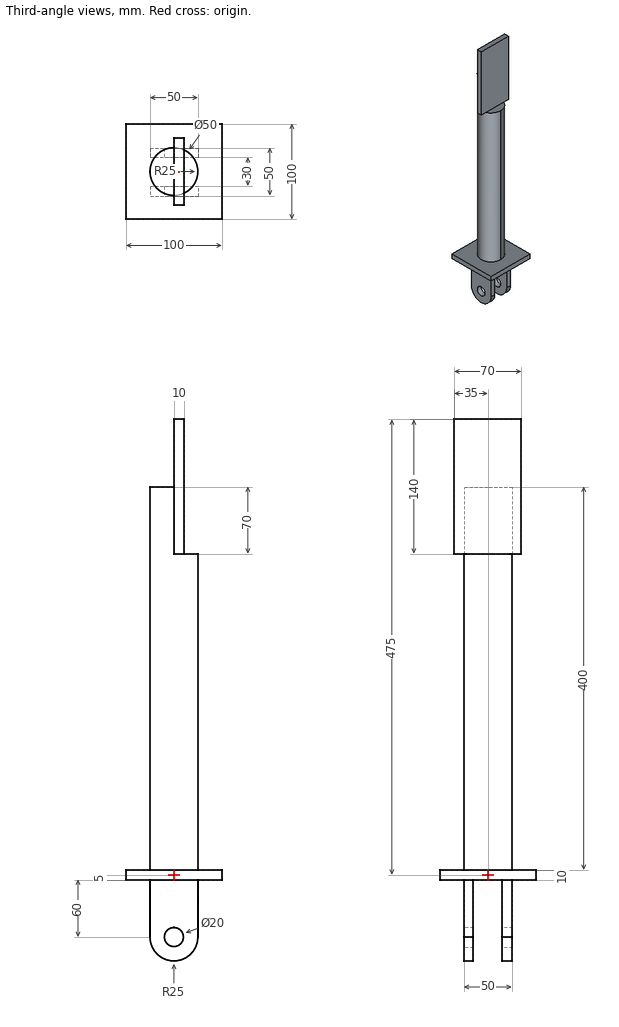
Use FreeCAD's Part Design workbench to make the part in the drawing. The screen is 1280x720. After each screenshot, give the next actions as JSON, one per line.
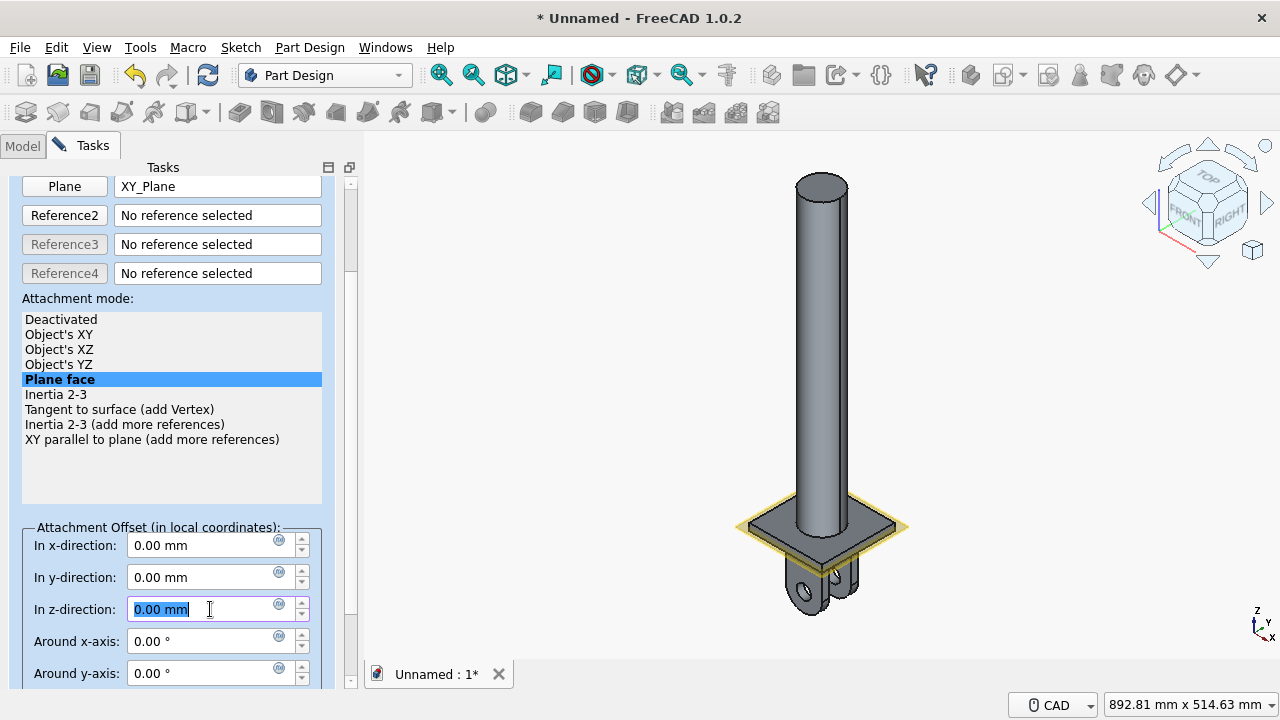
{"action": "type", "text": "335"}
{"action": "key", "text": "Tab"}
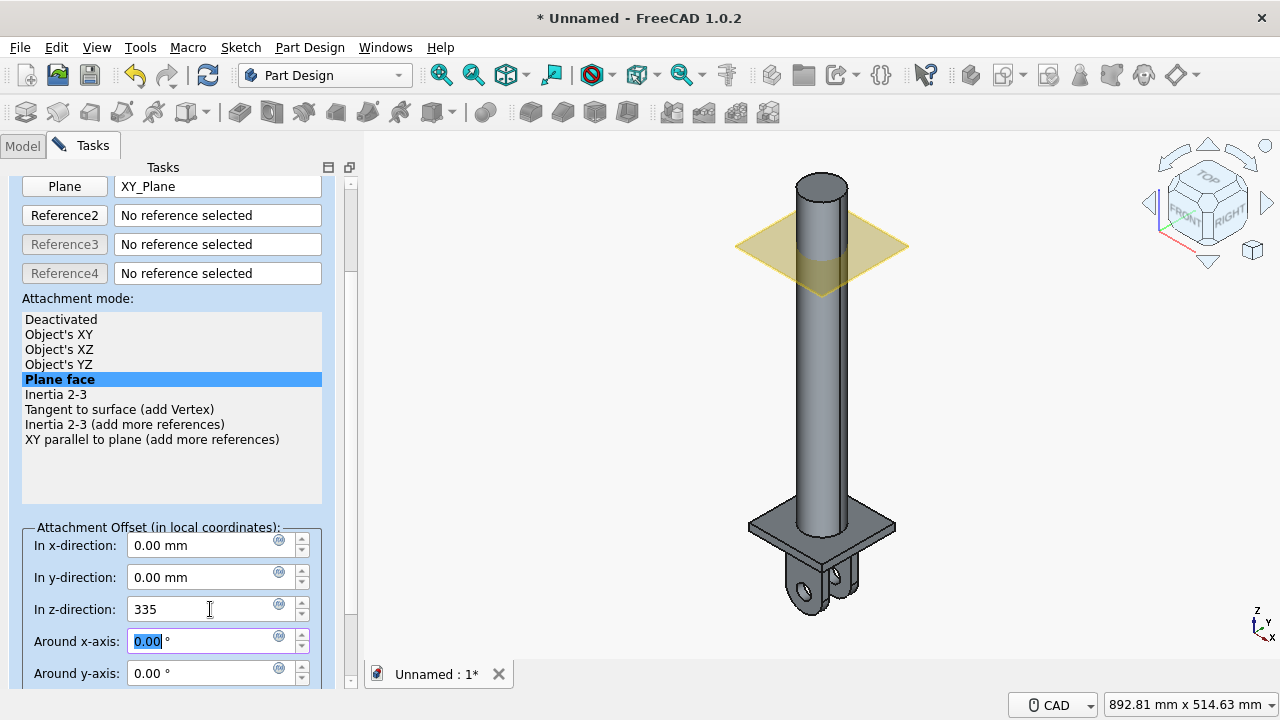
{"action": "scroll", "coordinate": [351, 432], "scroll_direction": "up", "scroll_amount": 3}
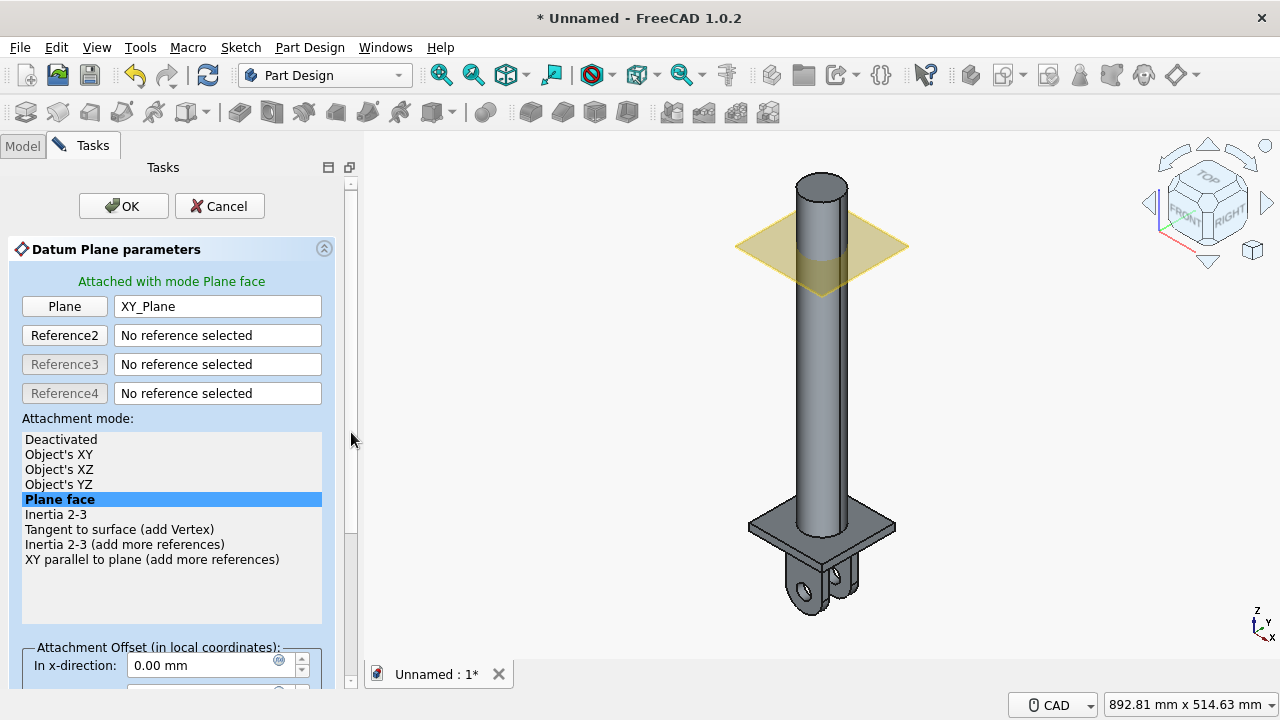
{"action": "left_click", "coordinate": [124, 206]}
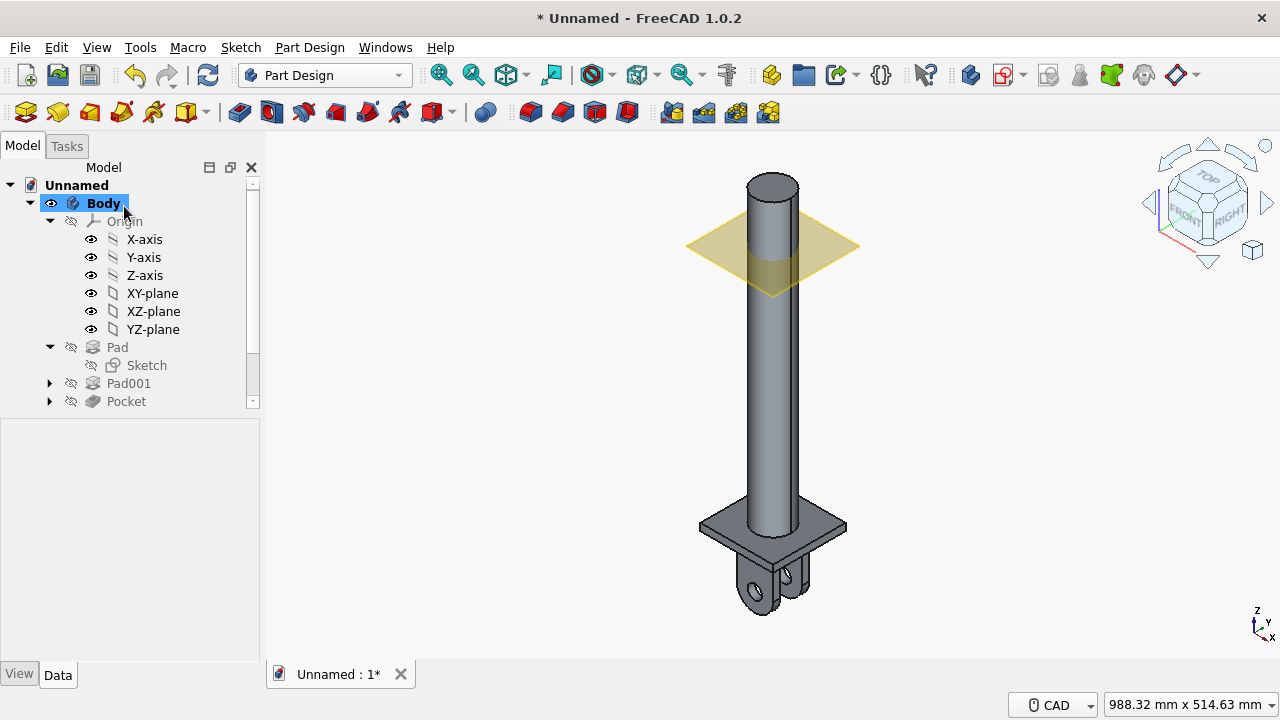
{"action": "scroll", "coordinate": [100, 289], "scroll_direction": "down", "scroll_amount": 3}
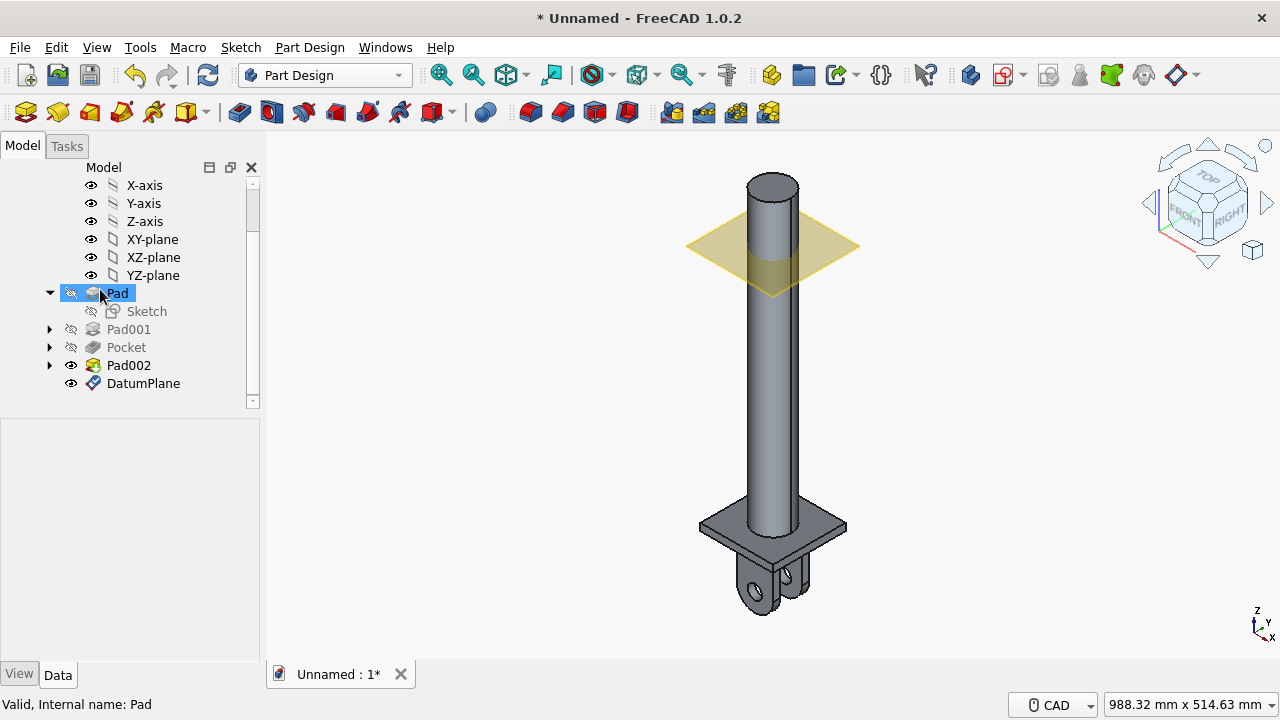
{"action": "left_click", "coordinate": [116, 383]}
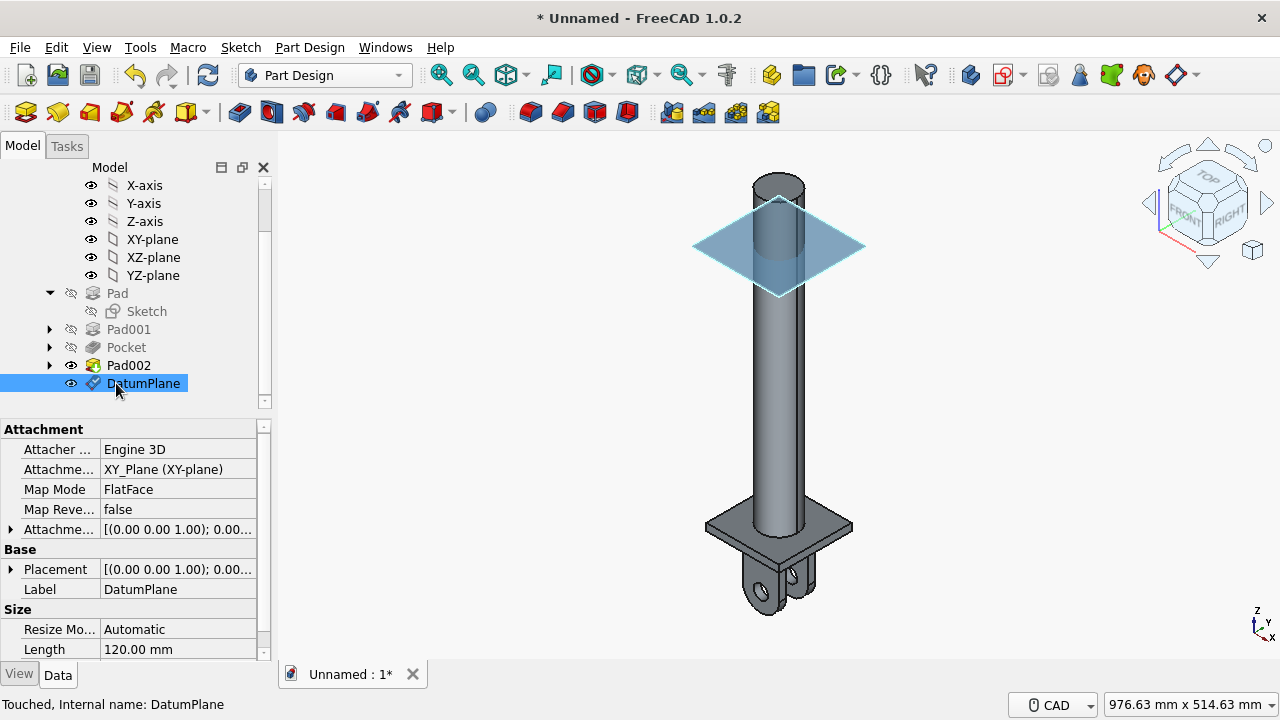
{"action": "left_click", "coordinate": [1004, 76]}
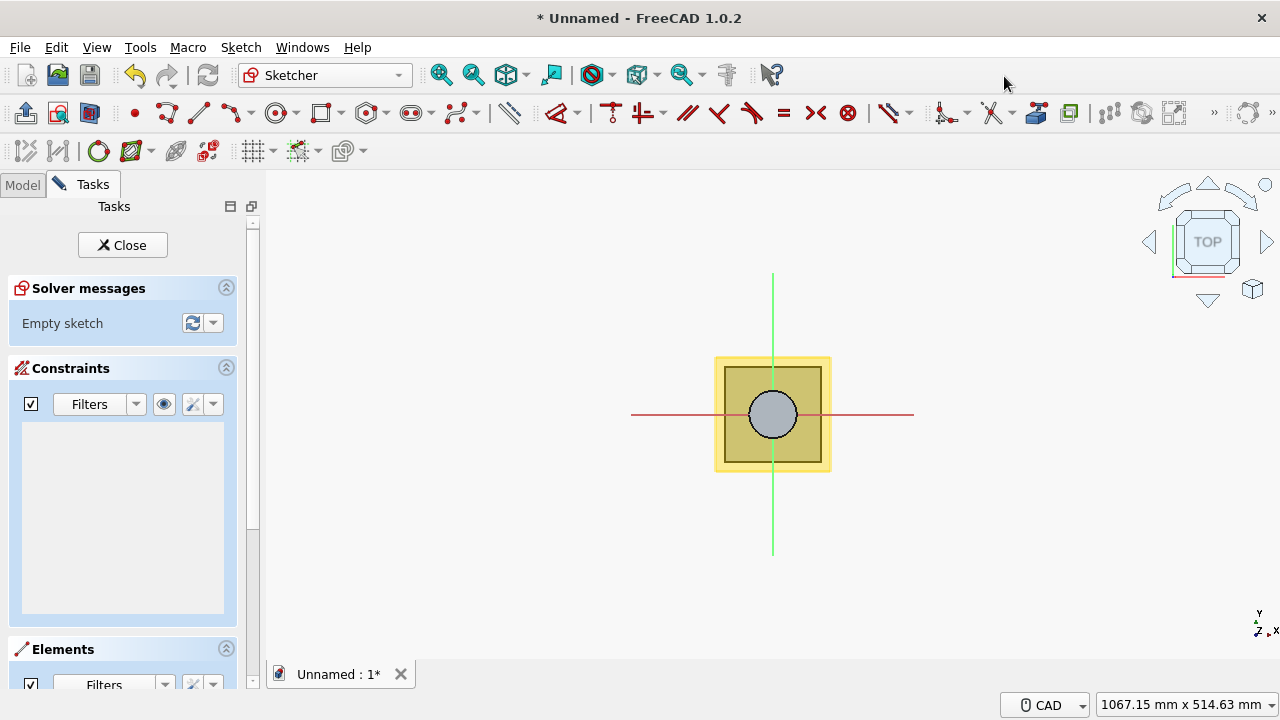
{"action": "key", "text": "q s"}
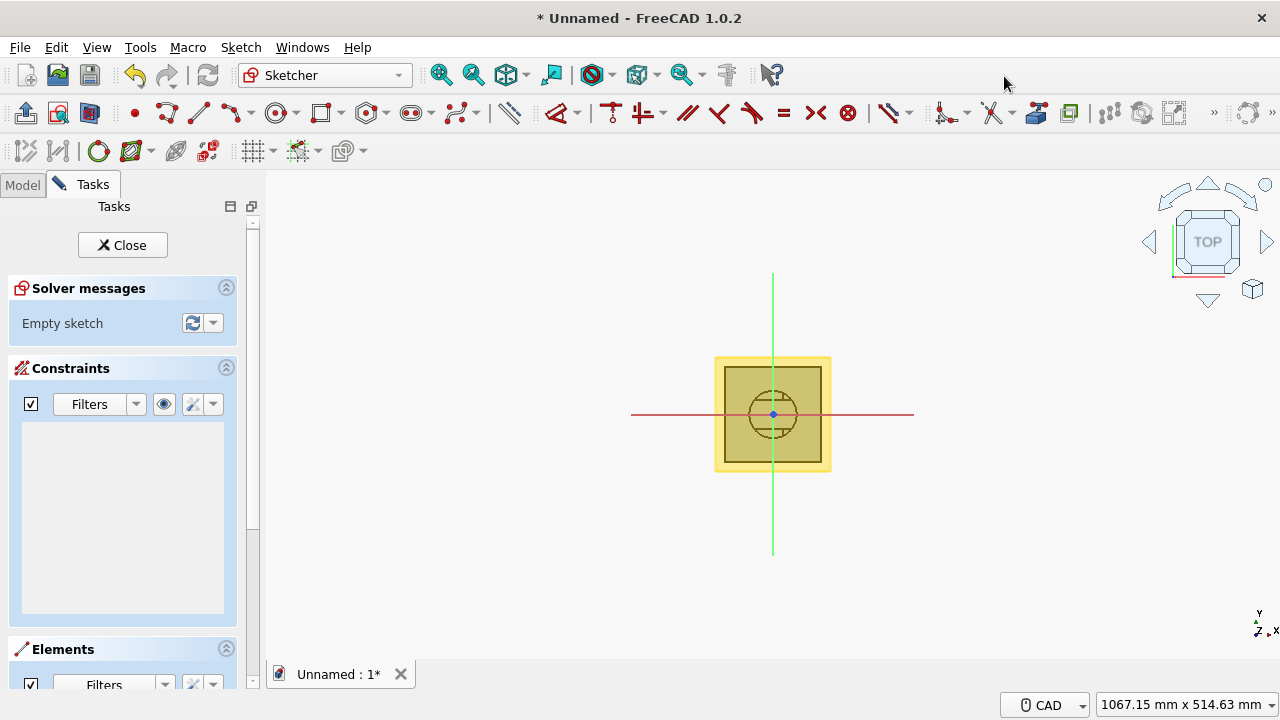
{"action": "scroll", "coordinate": [801, 414], "scroll_direction": "up", "scroll_amount": 9}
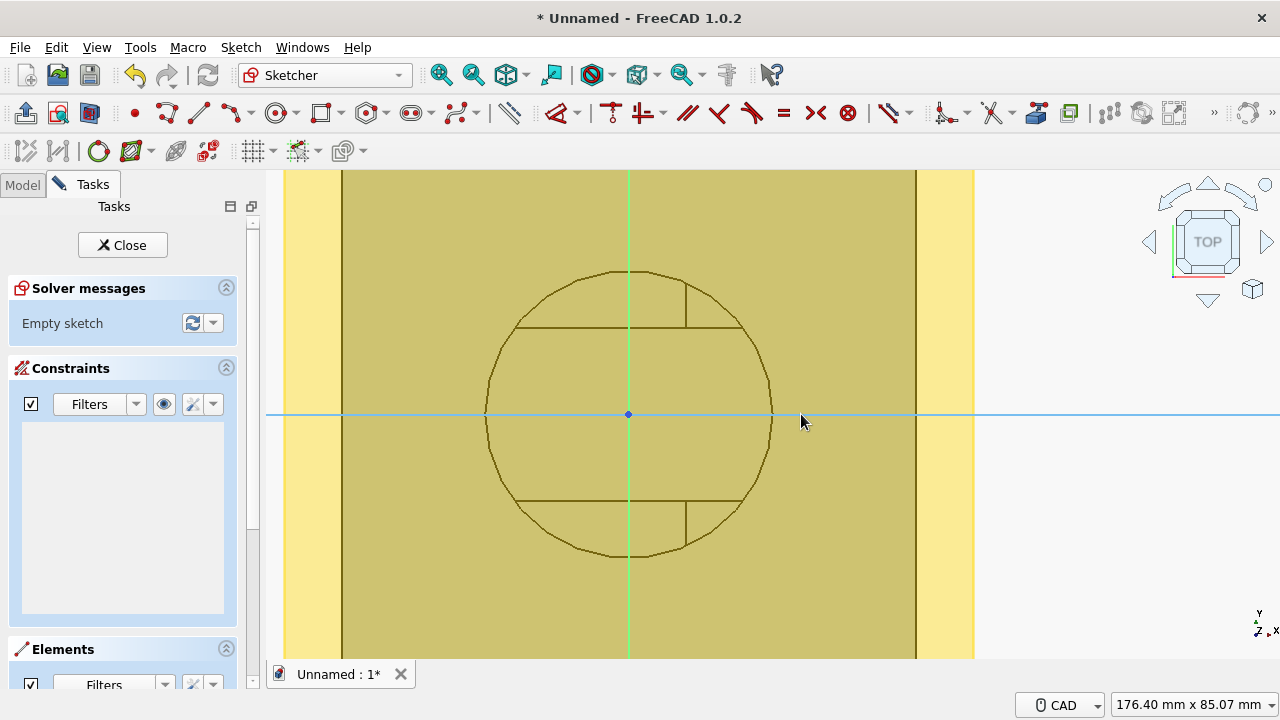
{"action": "key", "text": "g l"}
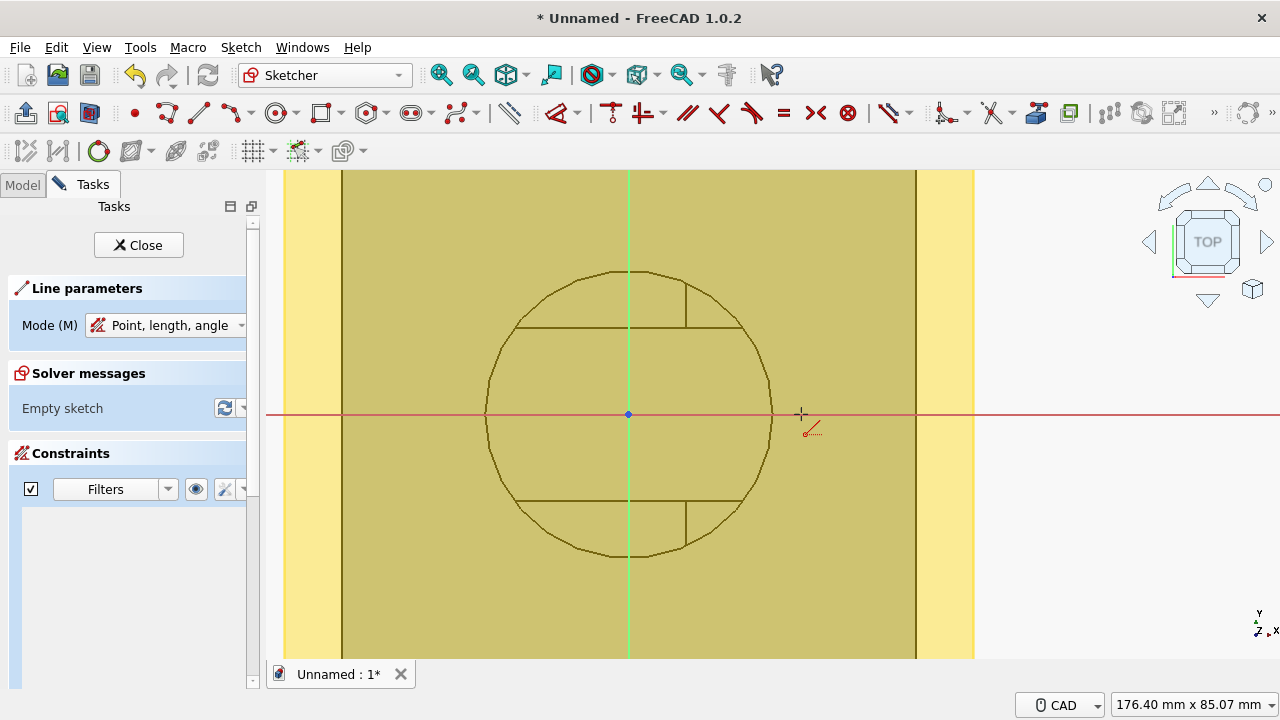
{"action": "left_click", "coordinate": [629, 271]}
{"action": "left_click", "coordinate": [638, 558]}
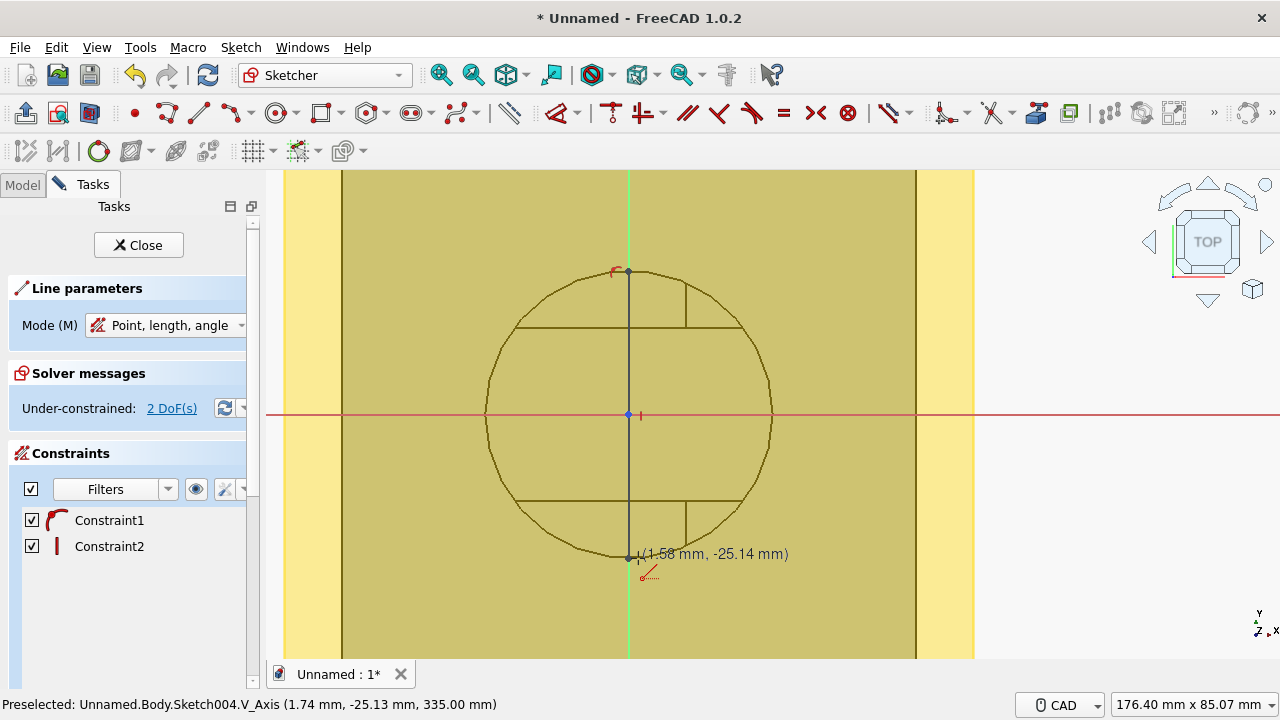
{"action": "key", "text": "g 3 a"}